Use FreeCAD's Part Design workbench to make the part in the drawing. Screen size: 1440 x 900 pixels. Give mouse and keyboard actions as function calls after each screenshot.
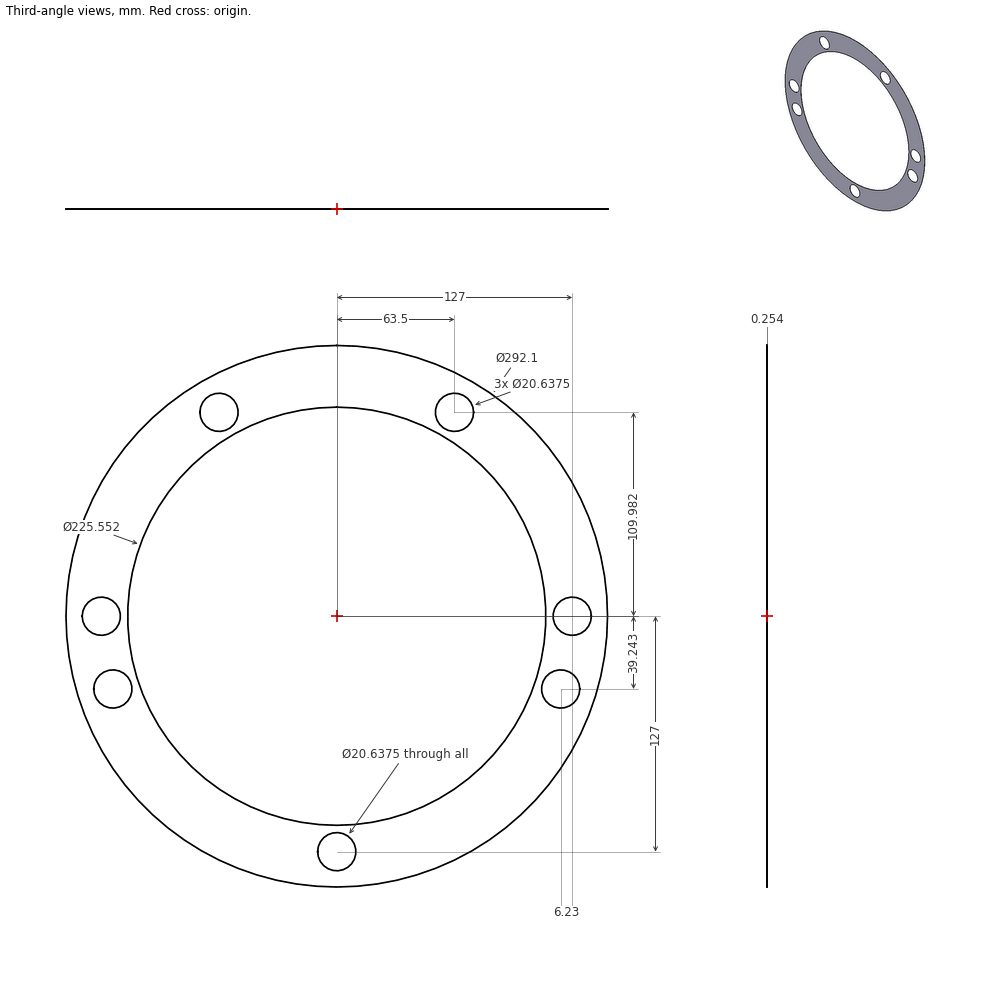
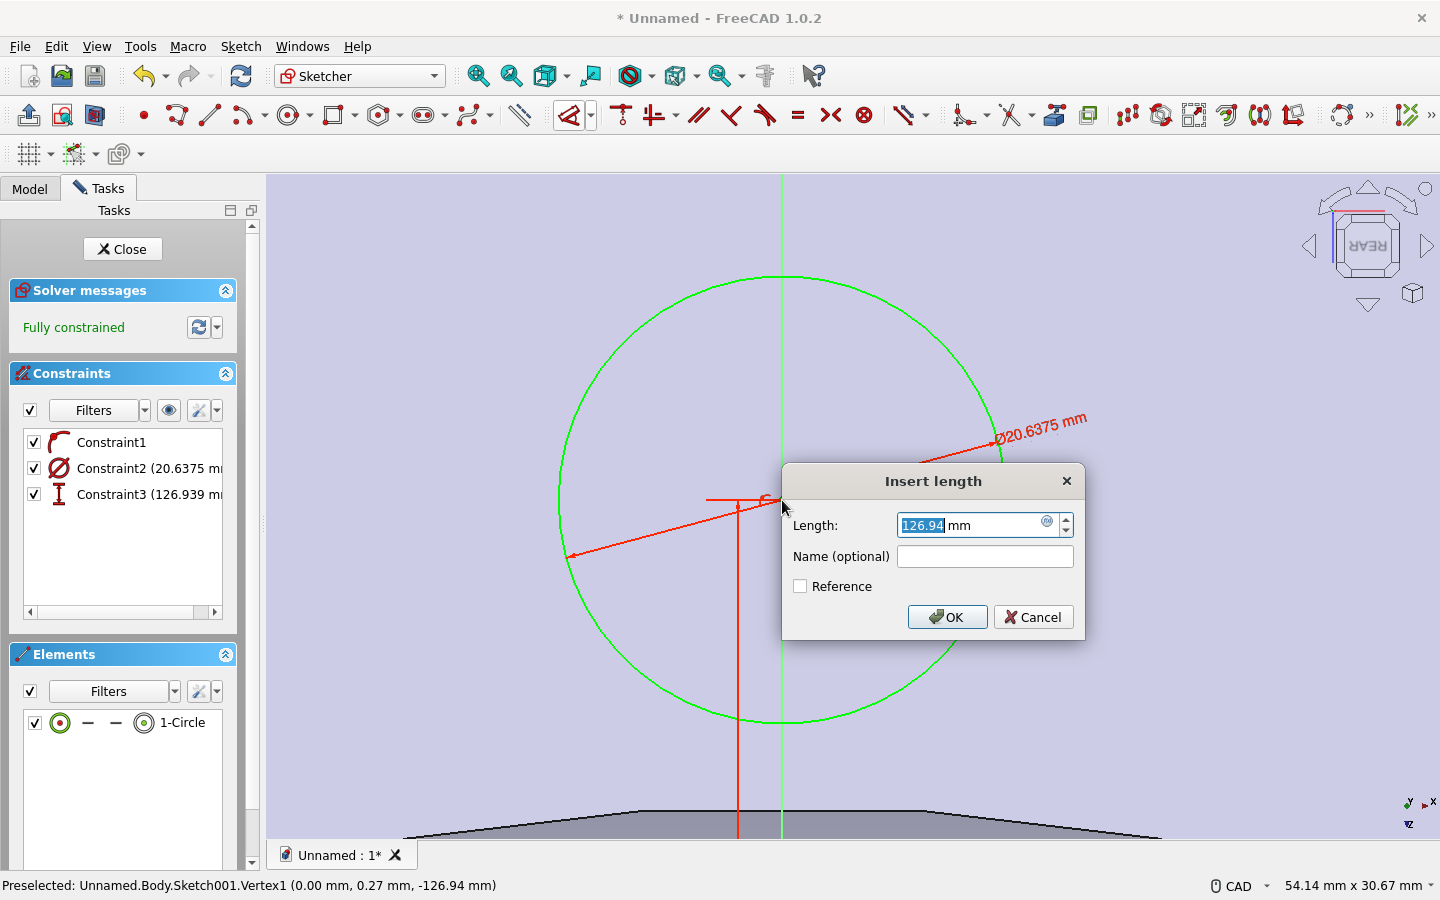
text(127)
key(Return)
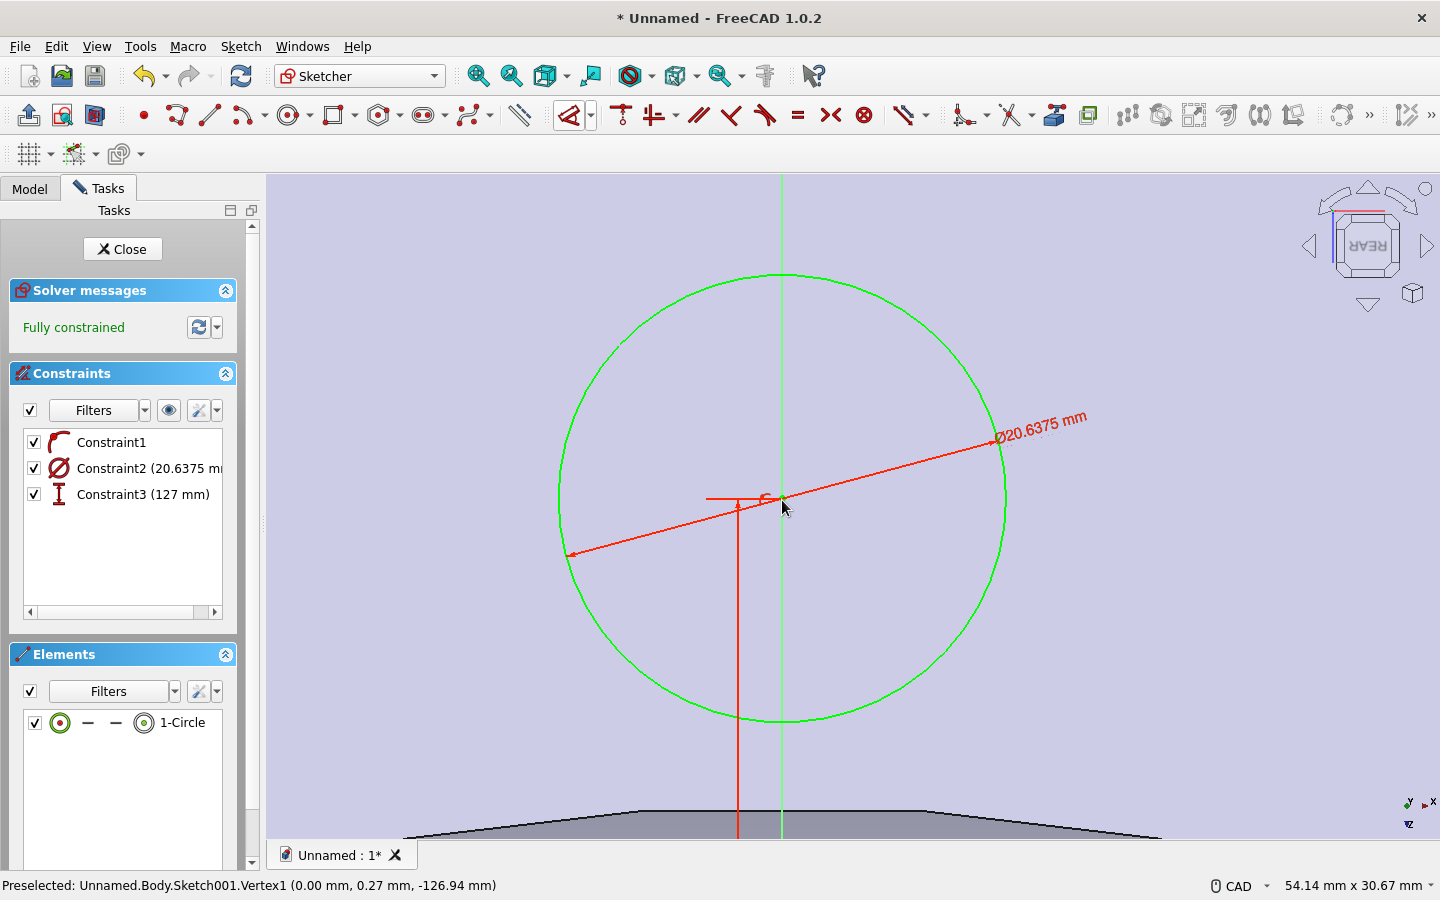
click(123, 249)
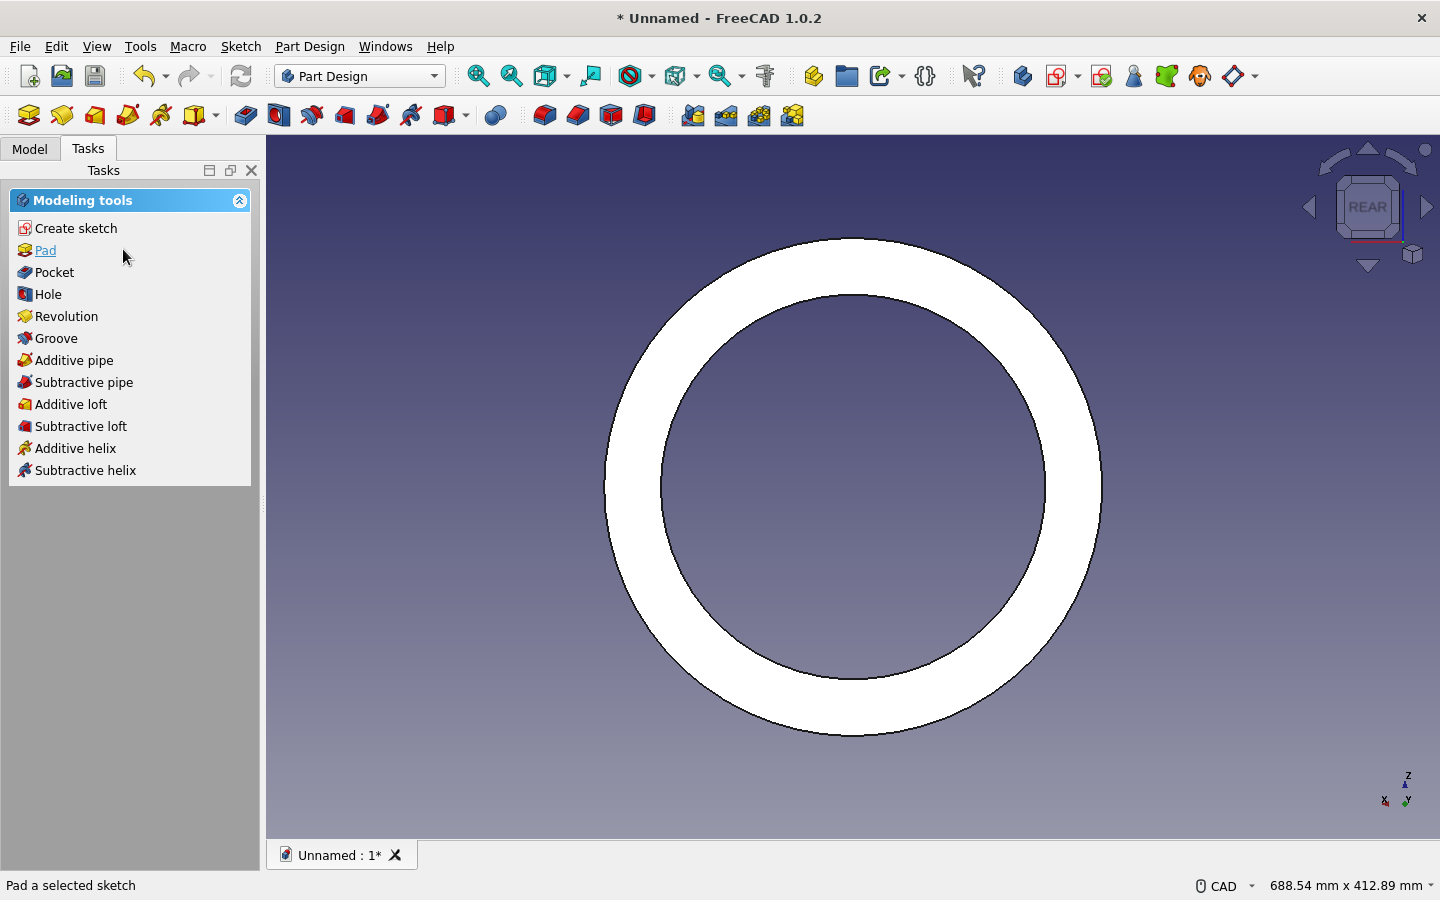
click(279, 116)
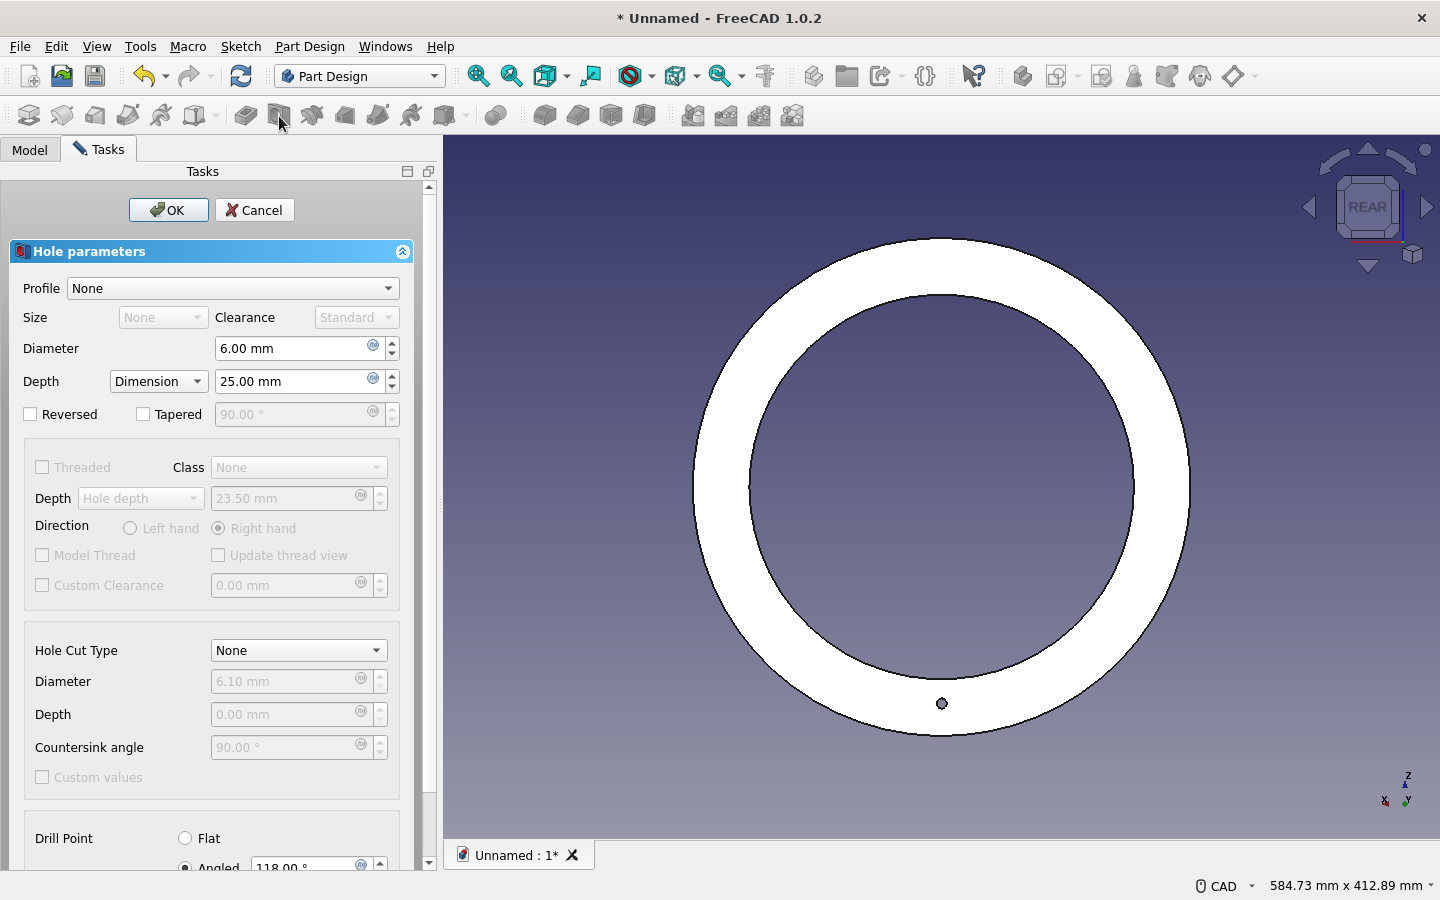
triple_click(300, 348)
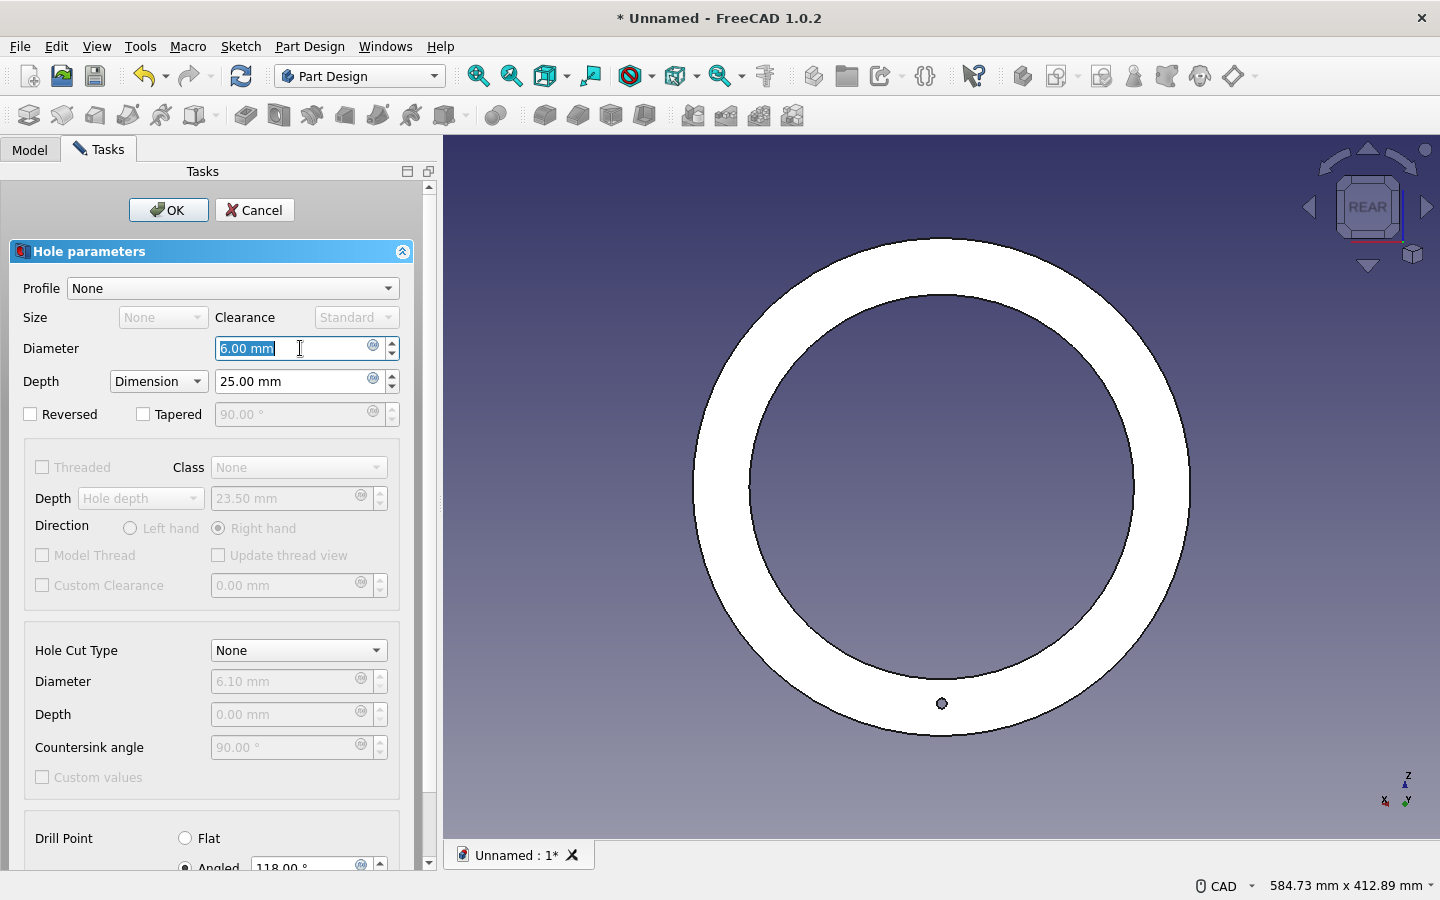
text(20.6375)
key(Tab)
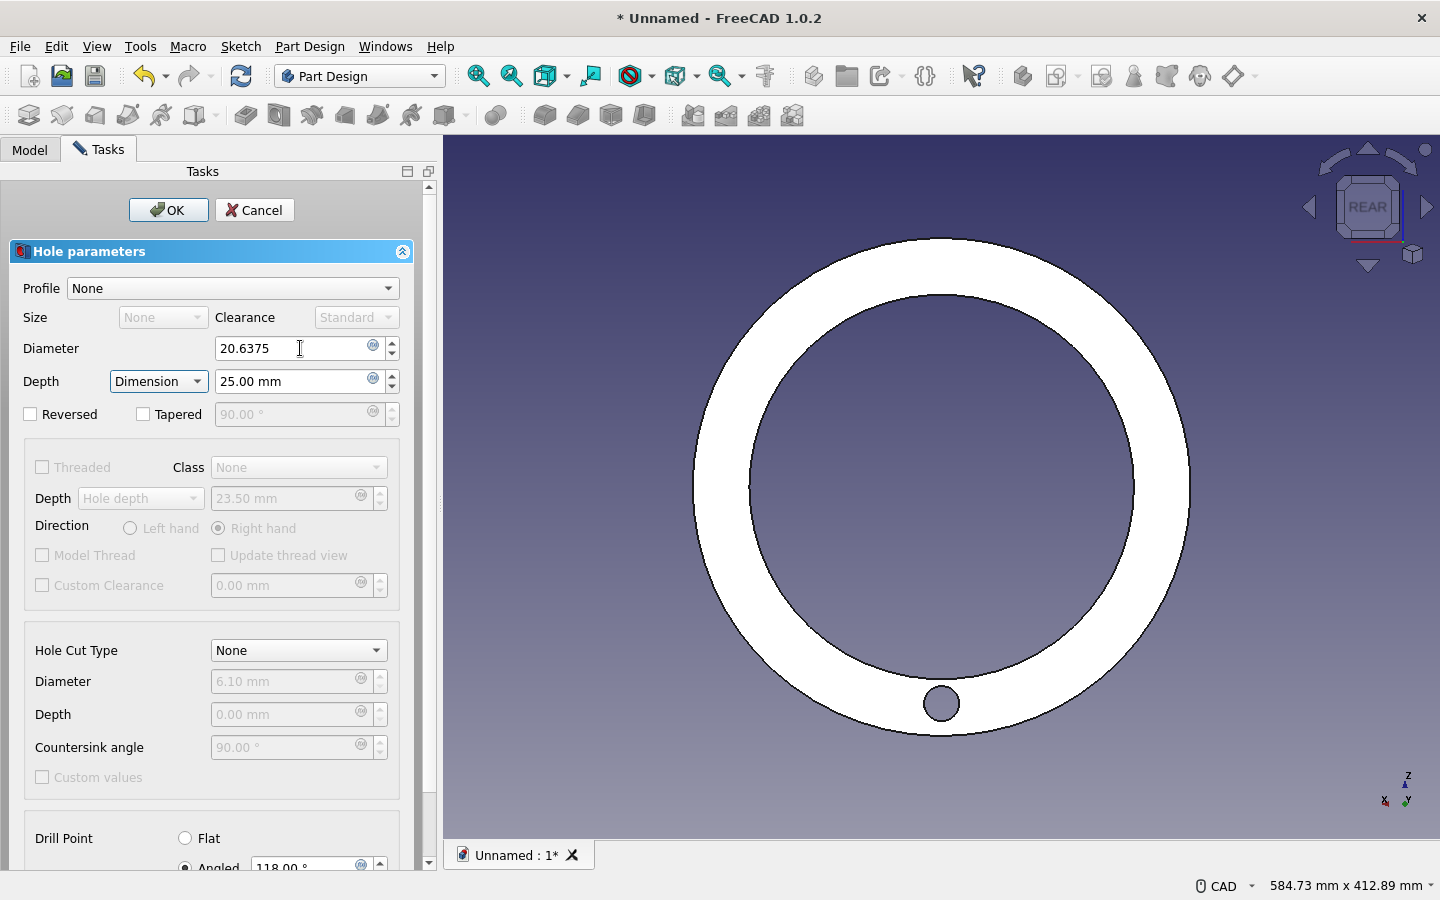
click(160, 382)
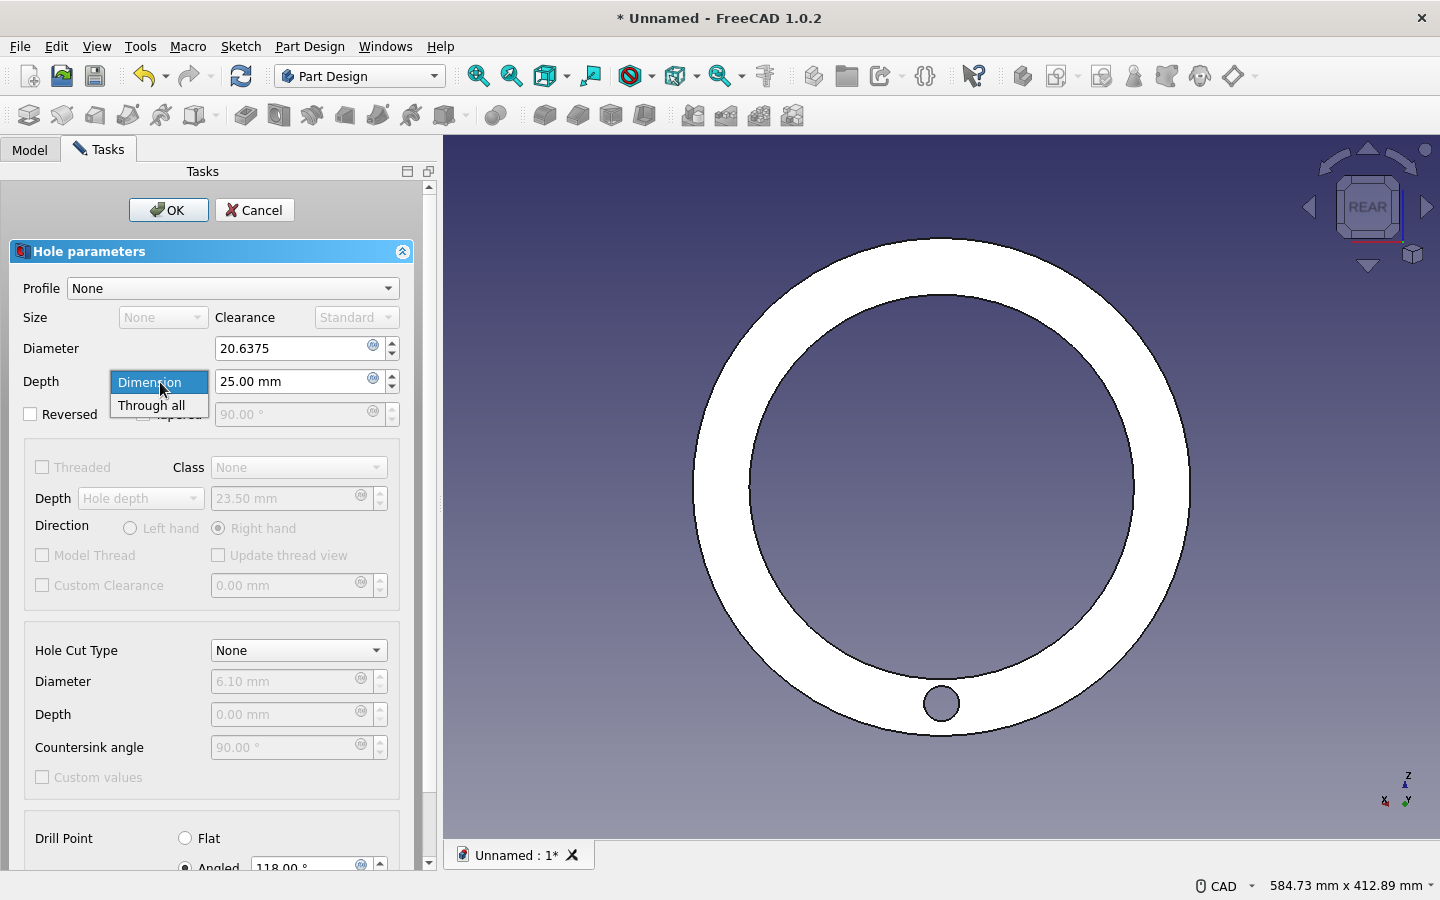
click(158, 406)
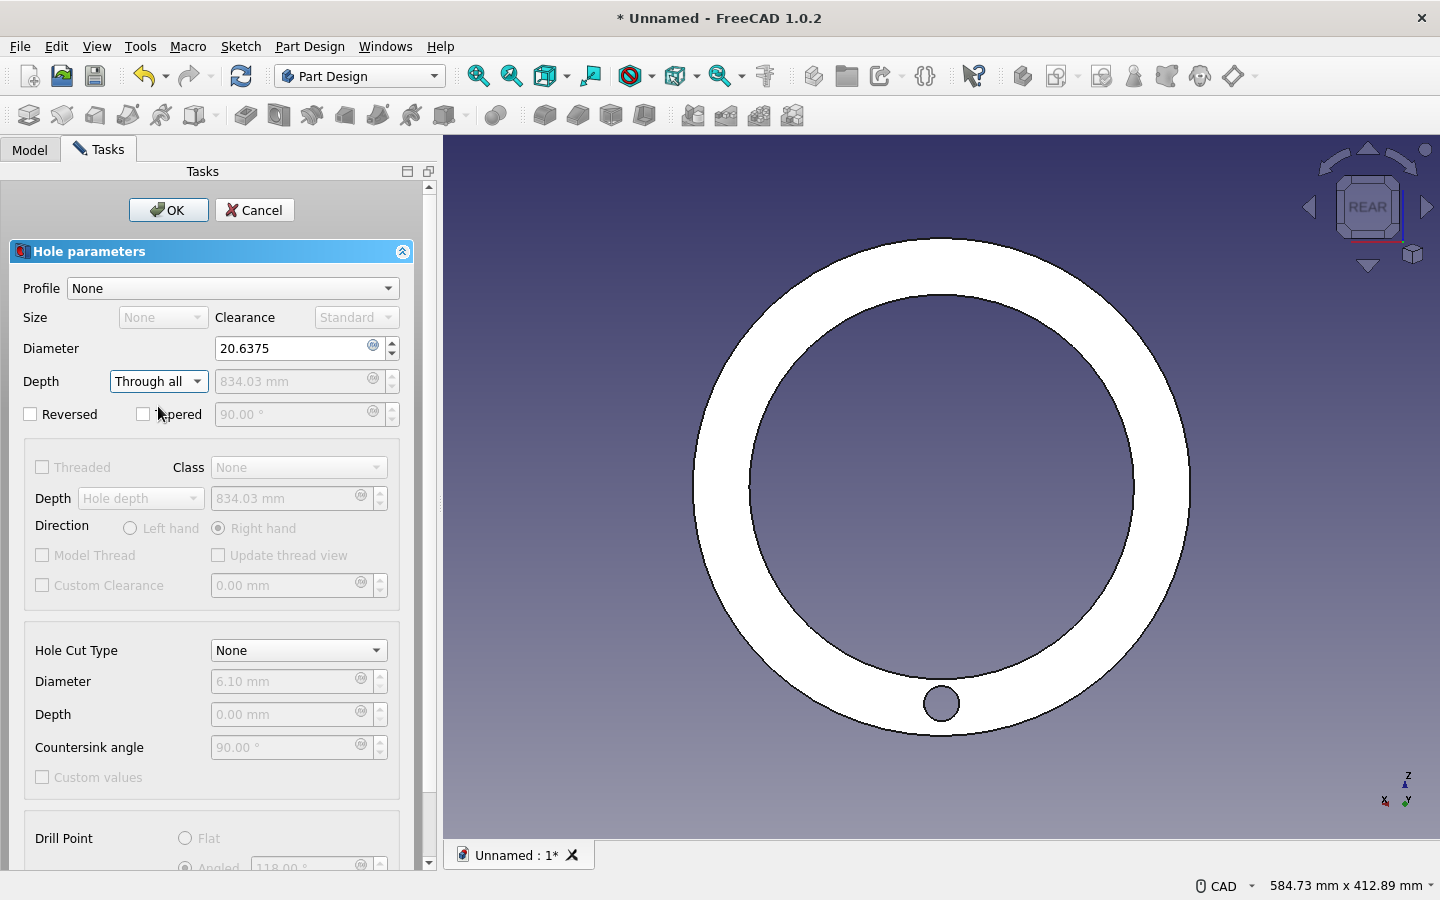
click(169, 210)